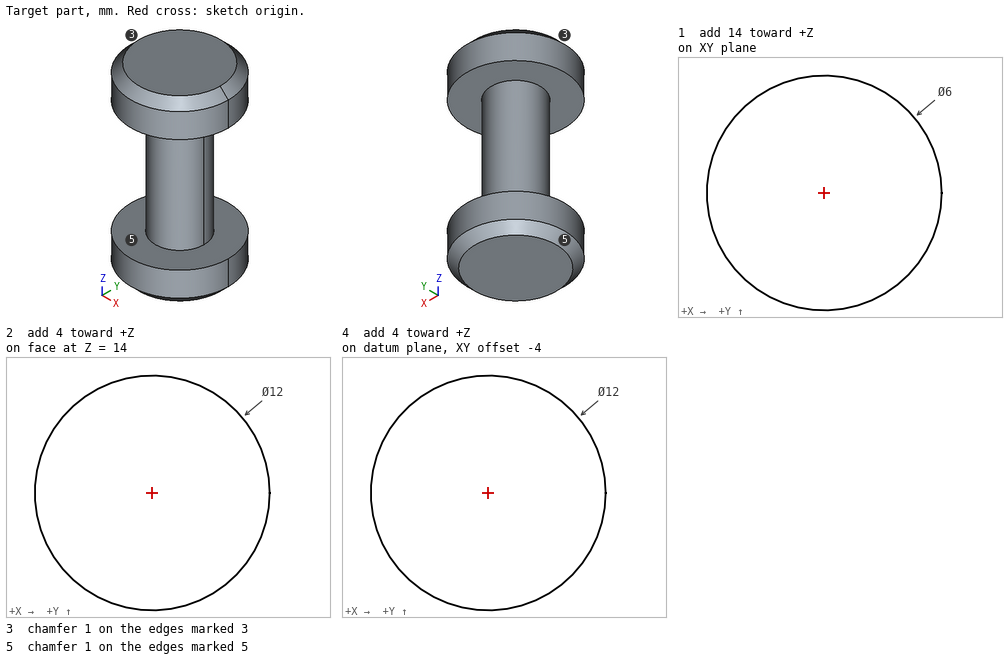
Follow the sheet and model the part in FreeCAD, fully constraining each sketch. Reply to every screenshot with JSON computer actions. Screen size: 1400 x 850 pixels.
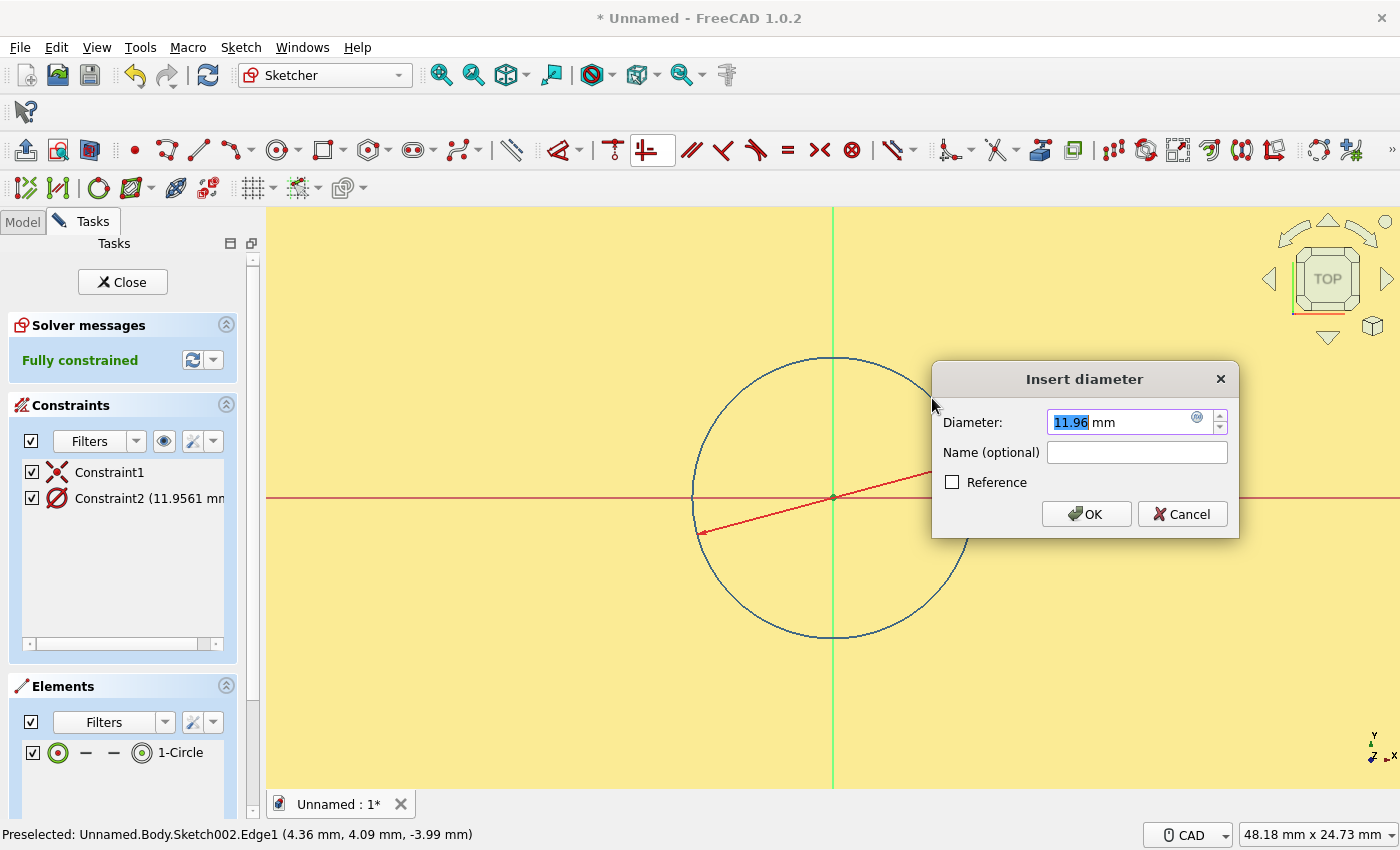
{"action": "type", "text": "12"}
{"action": "key", "text": "Return"}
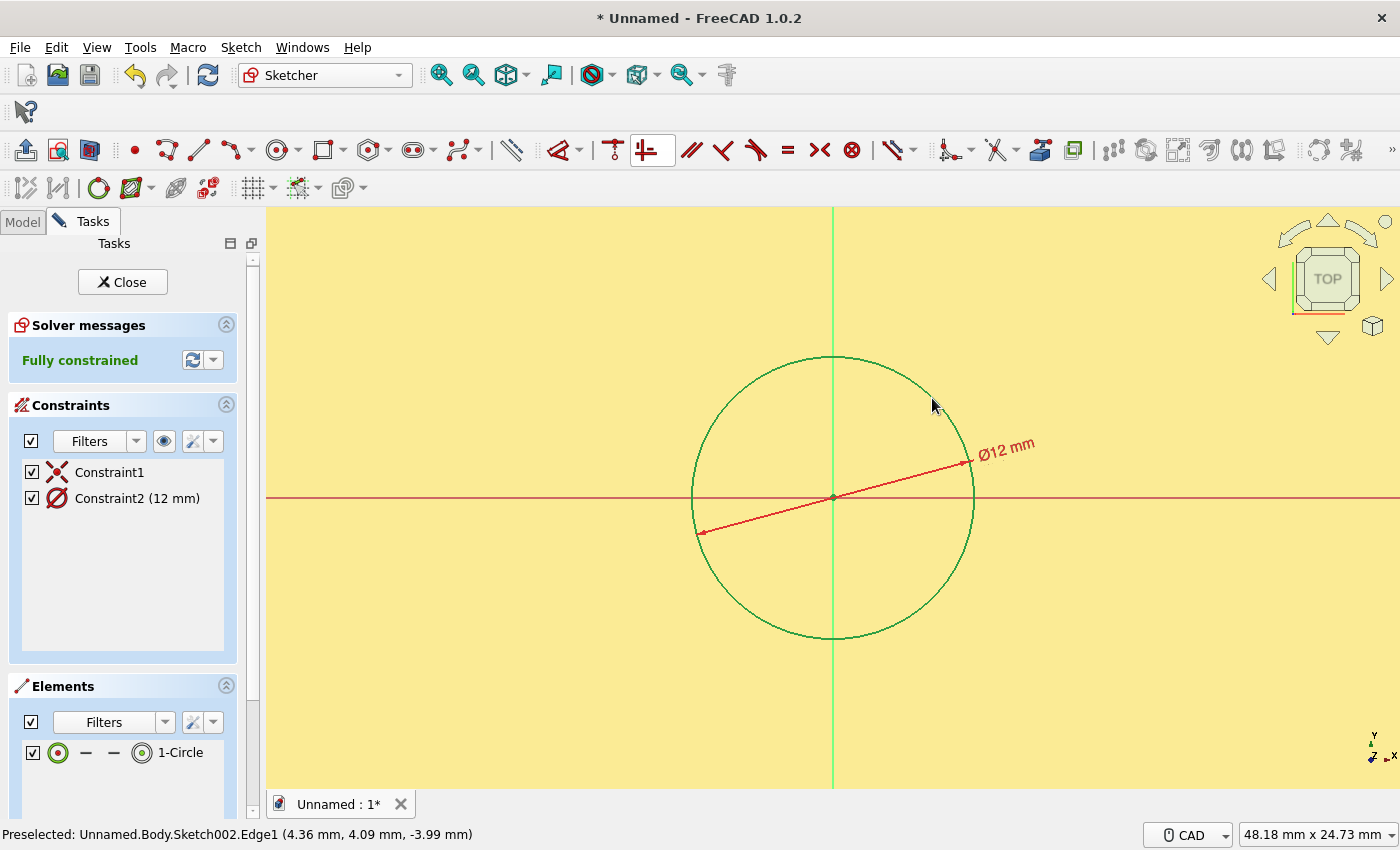
{"action": "left_click", "coordinate": [123, 282]}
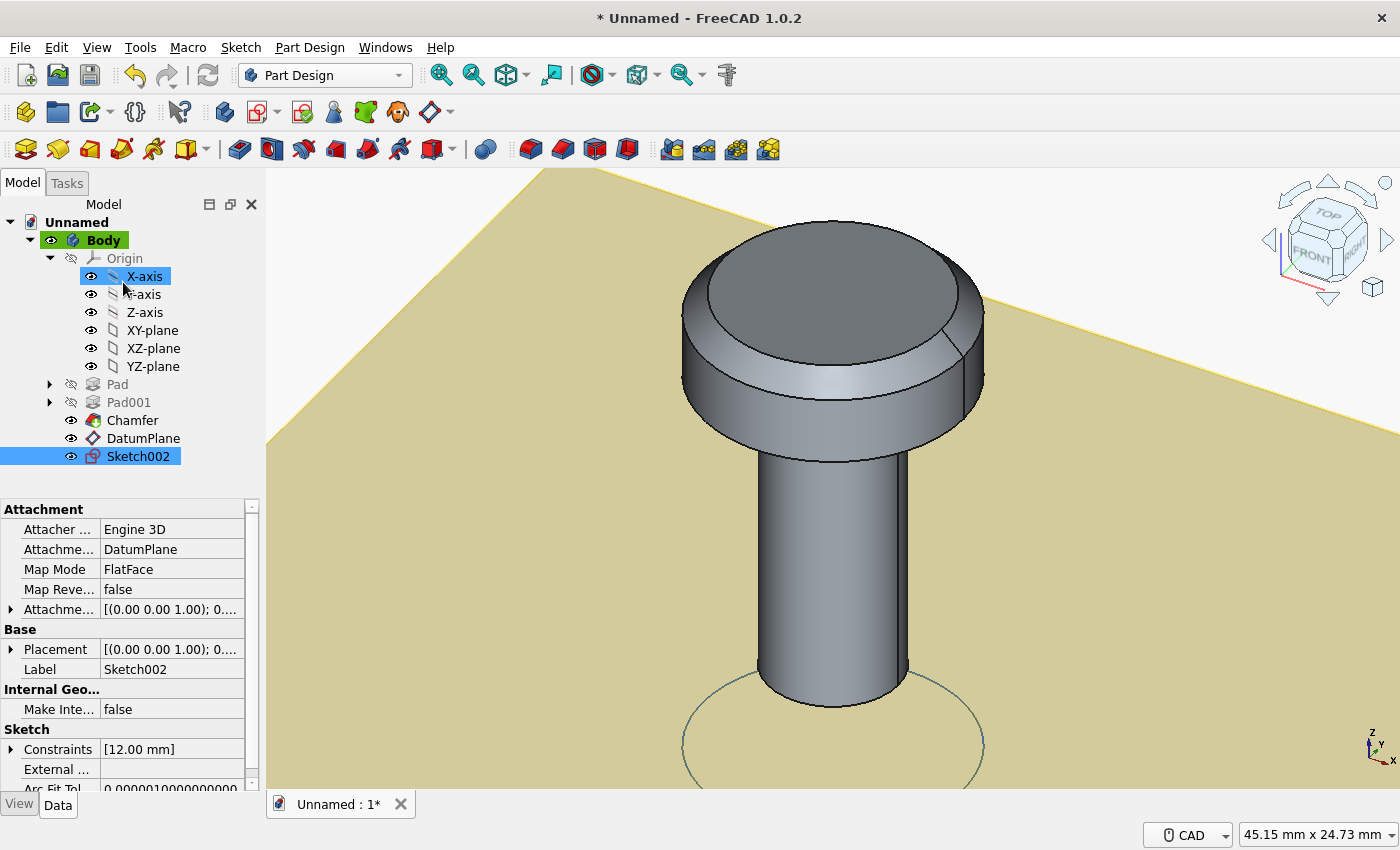
{"action": "left_click", "coordinate": [26, 150]}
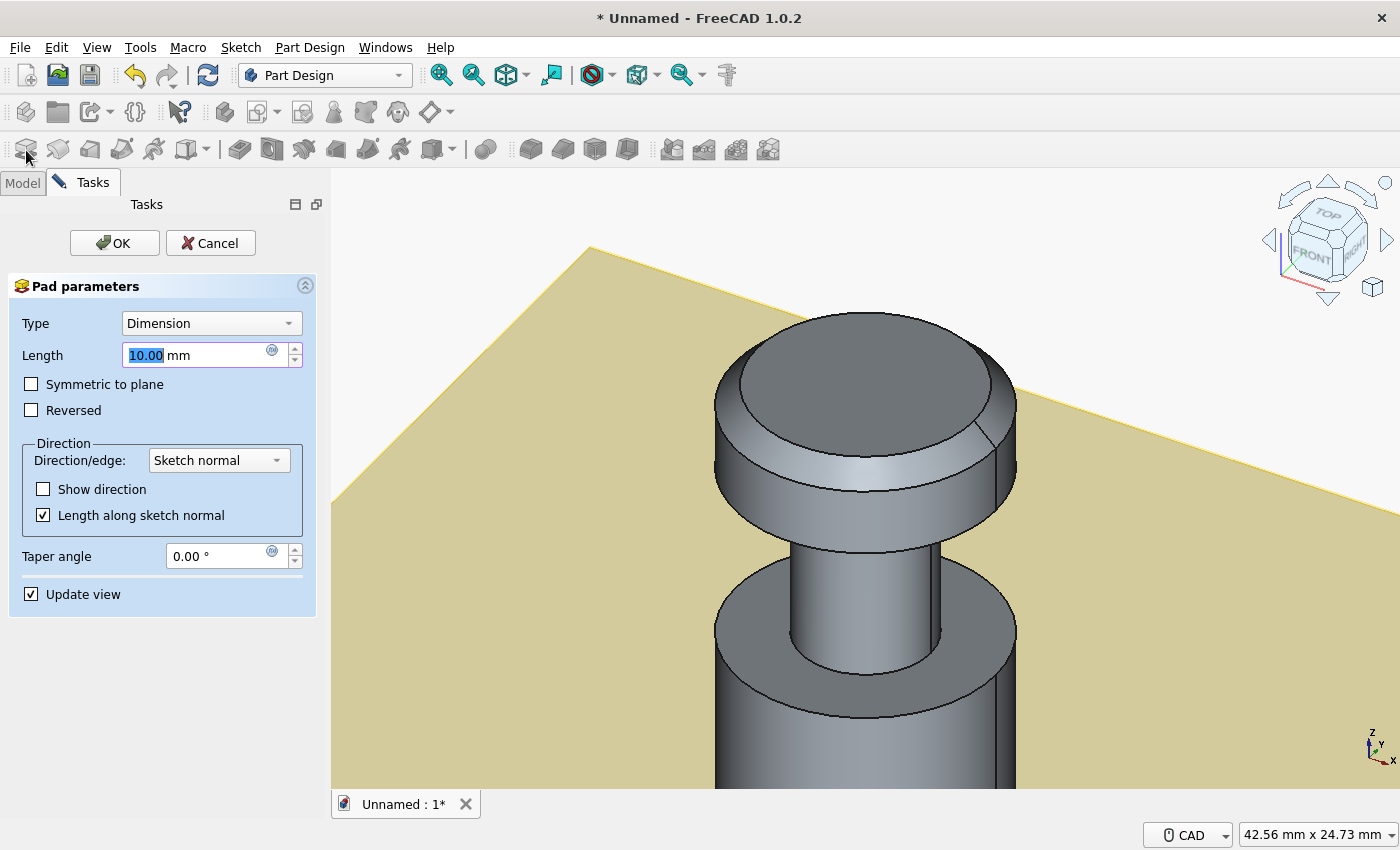
{"action": "type", "text": "4"}
{"action": "key", "text": "Tab"}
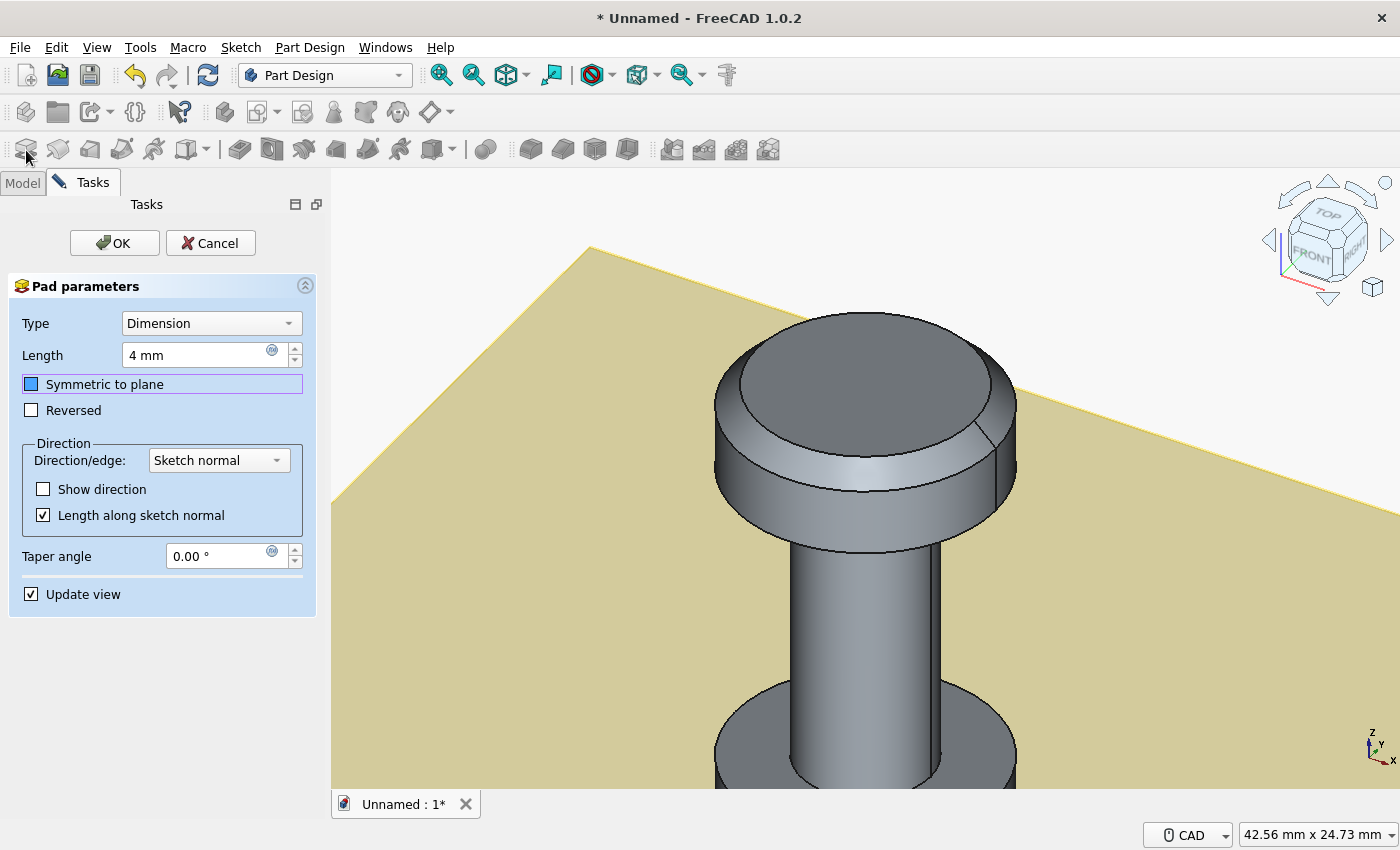
{"action": "left_click", "coordinate": [115, 243]}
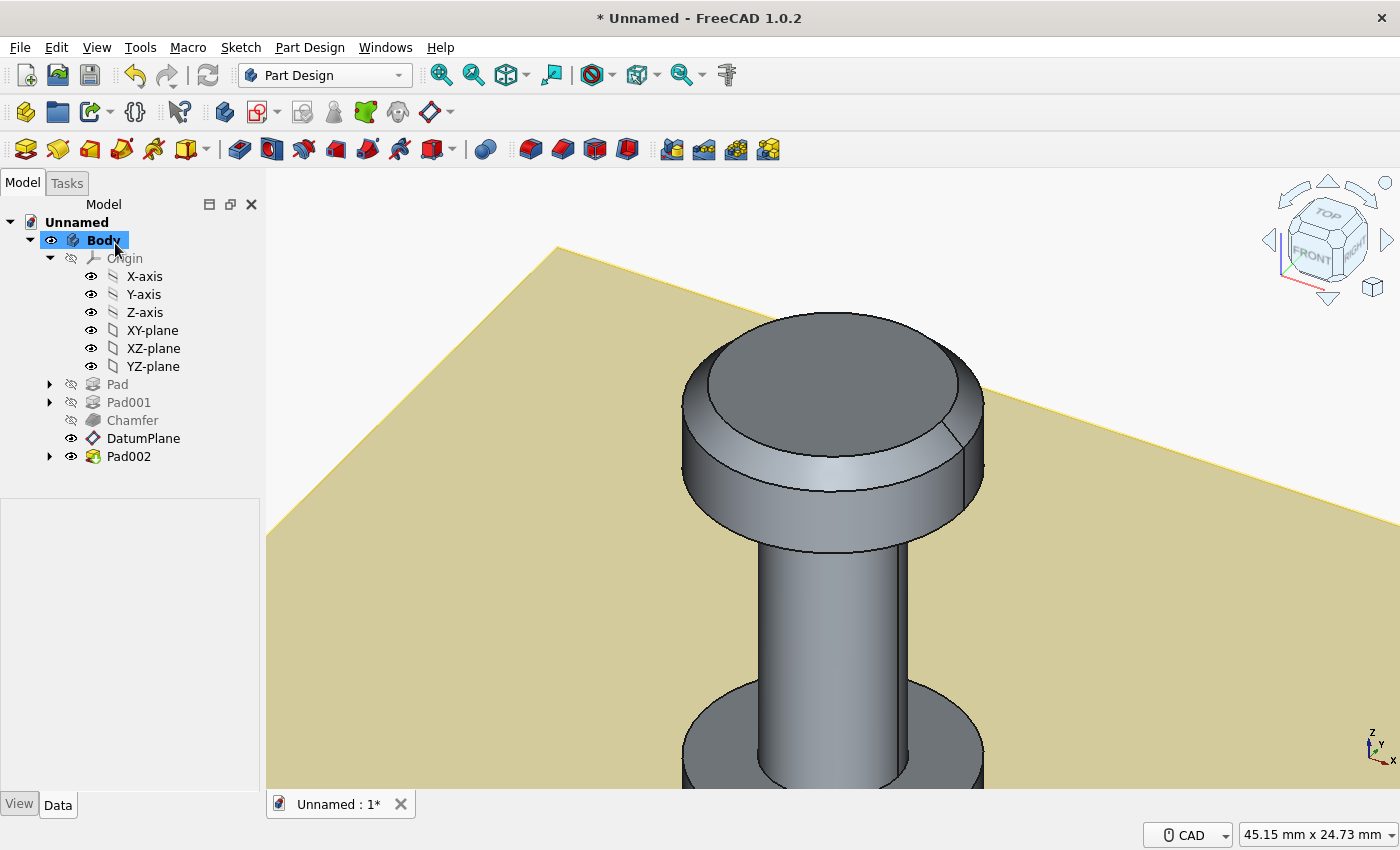
{"action": "left_click", "coordinate": [116, 438]}
{"action": "key", "text": "space"}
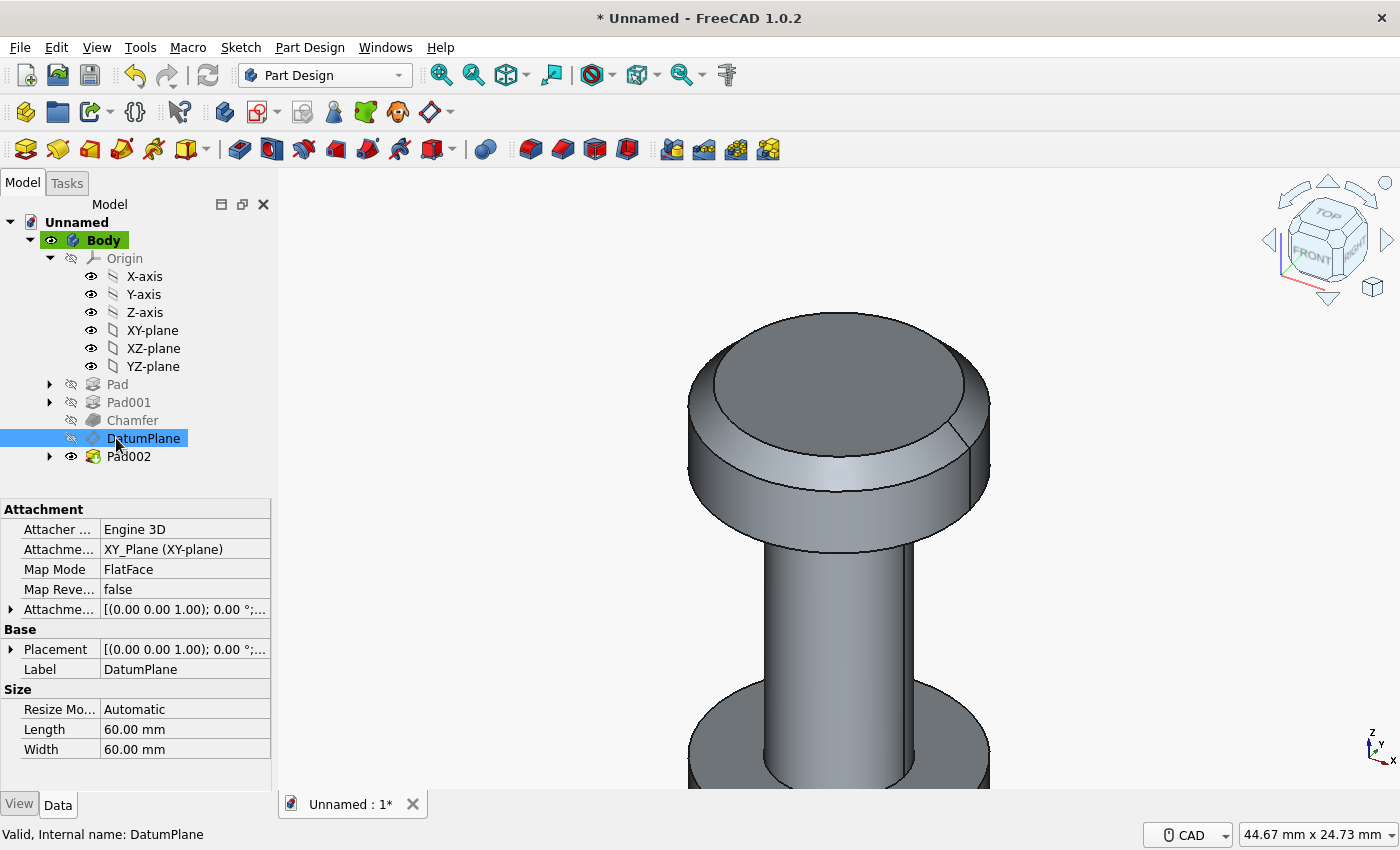
{"action": "key", "text": "v f"}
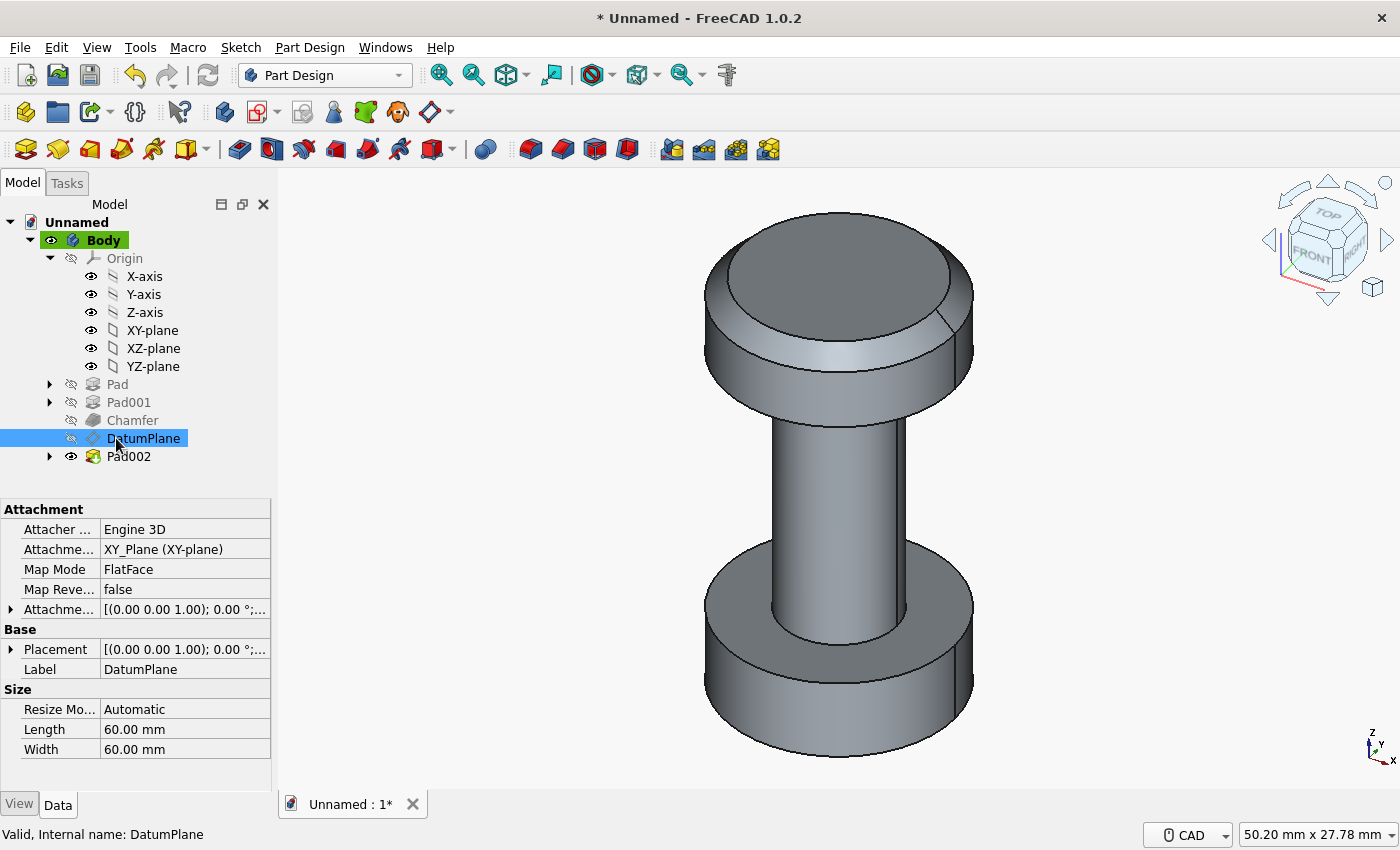
{"action": "key", "text": "0"}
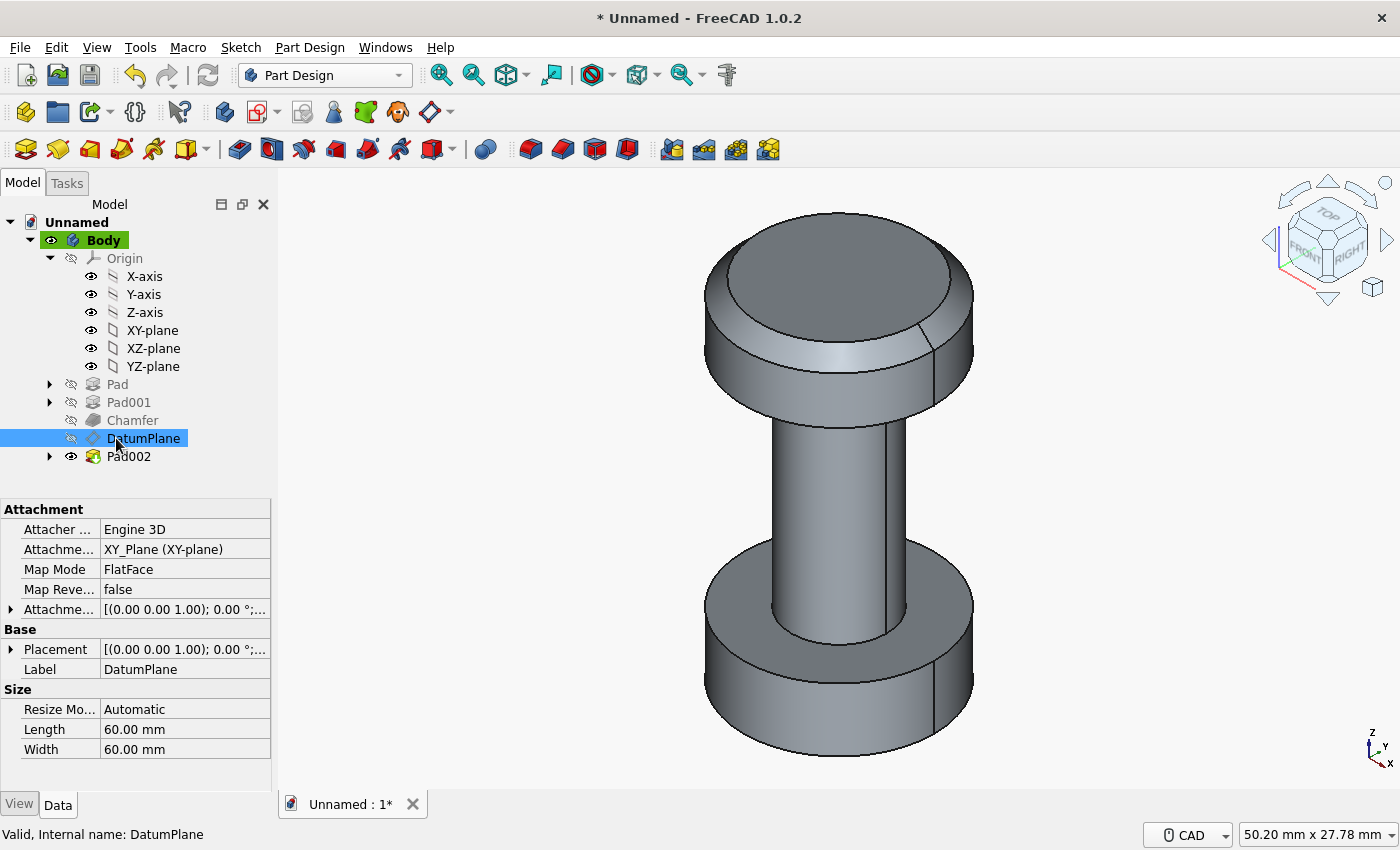
{"action": "key", "text": "v f"}